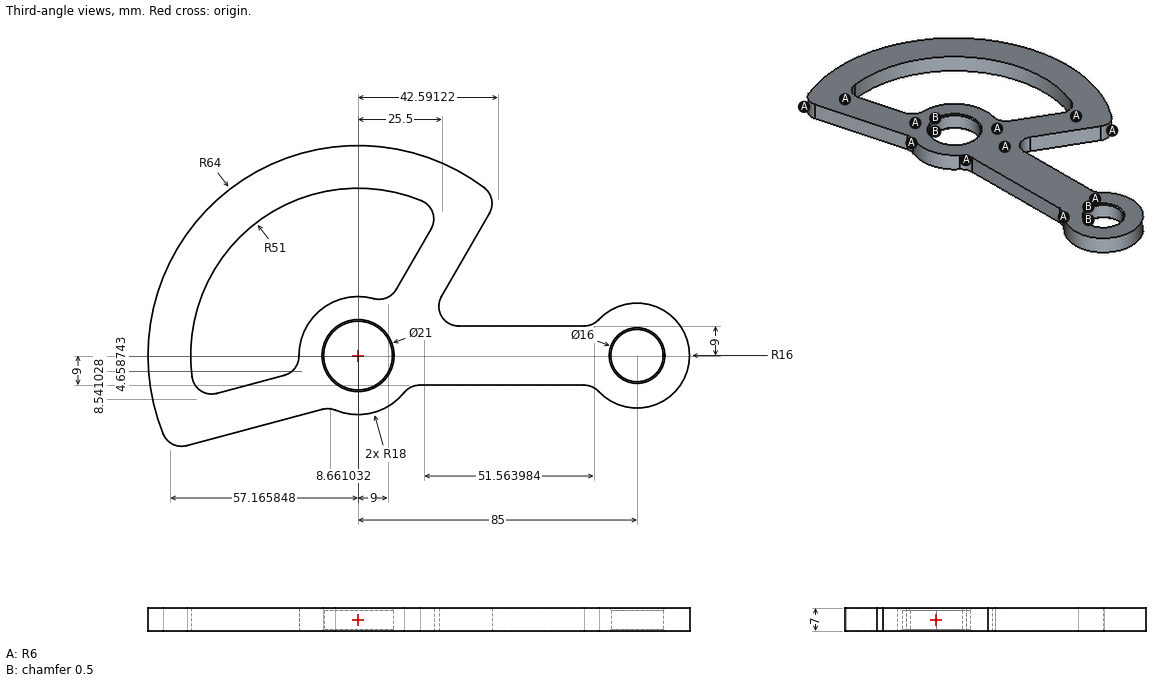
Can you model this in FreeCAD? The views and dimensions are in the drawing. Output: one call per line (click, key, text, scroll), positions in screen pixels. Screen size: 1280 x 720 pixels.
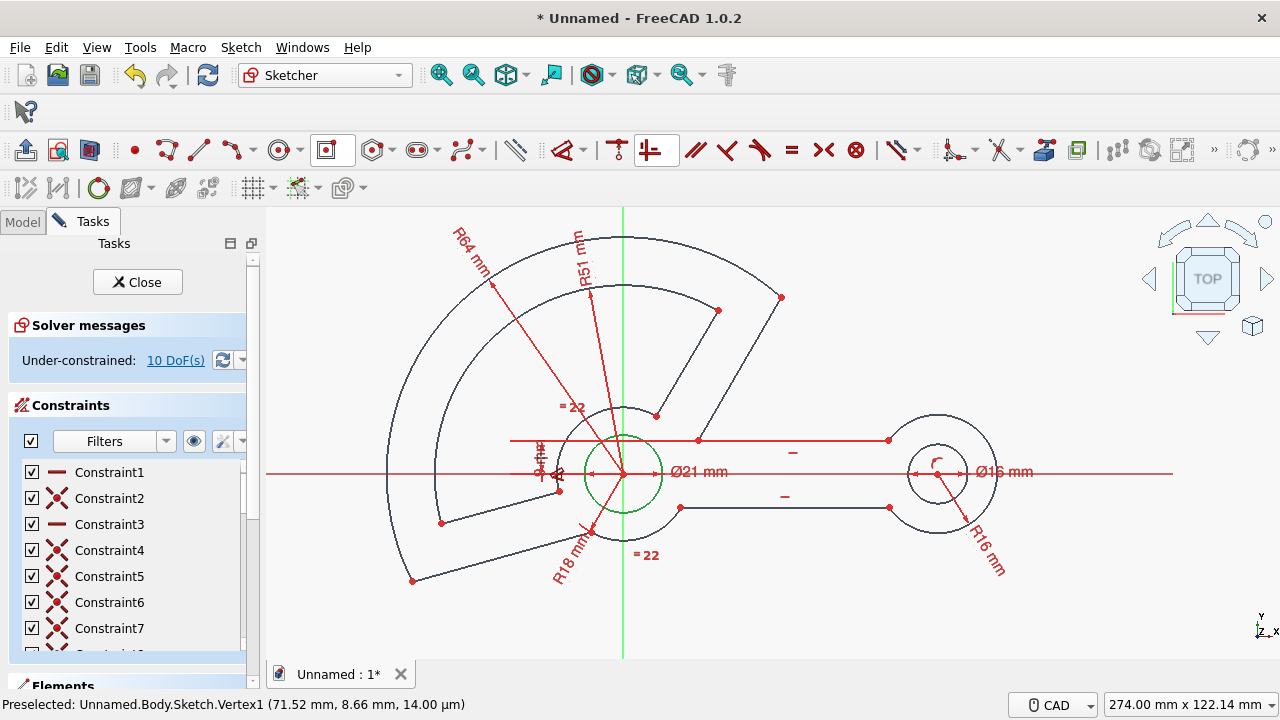
click(681, 508)
click(715, 491)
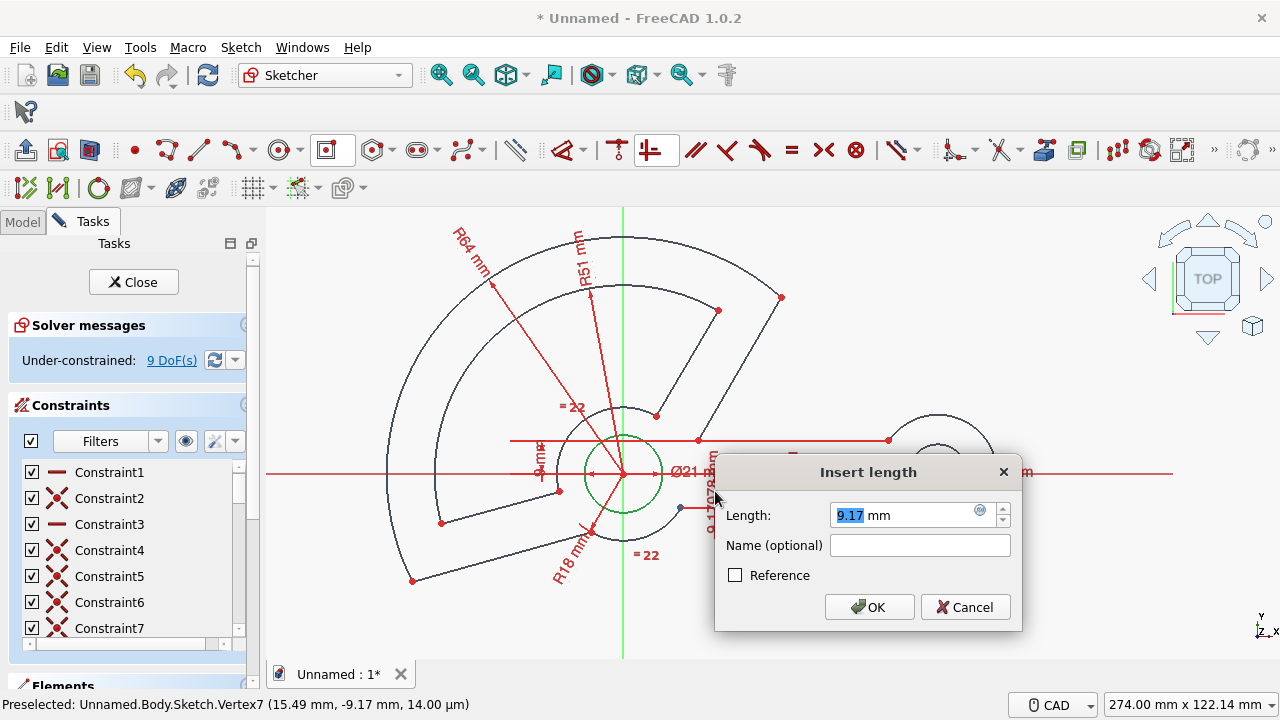
text(9)
key(Return)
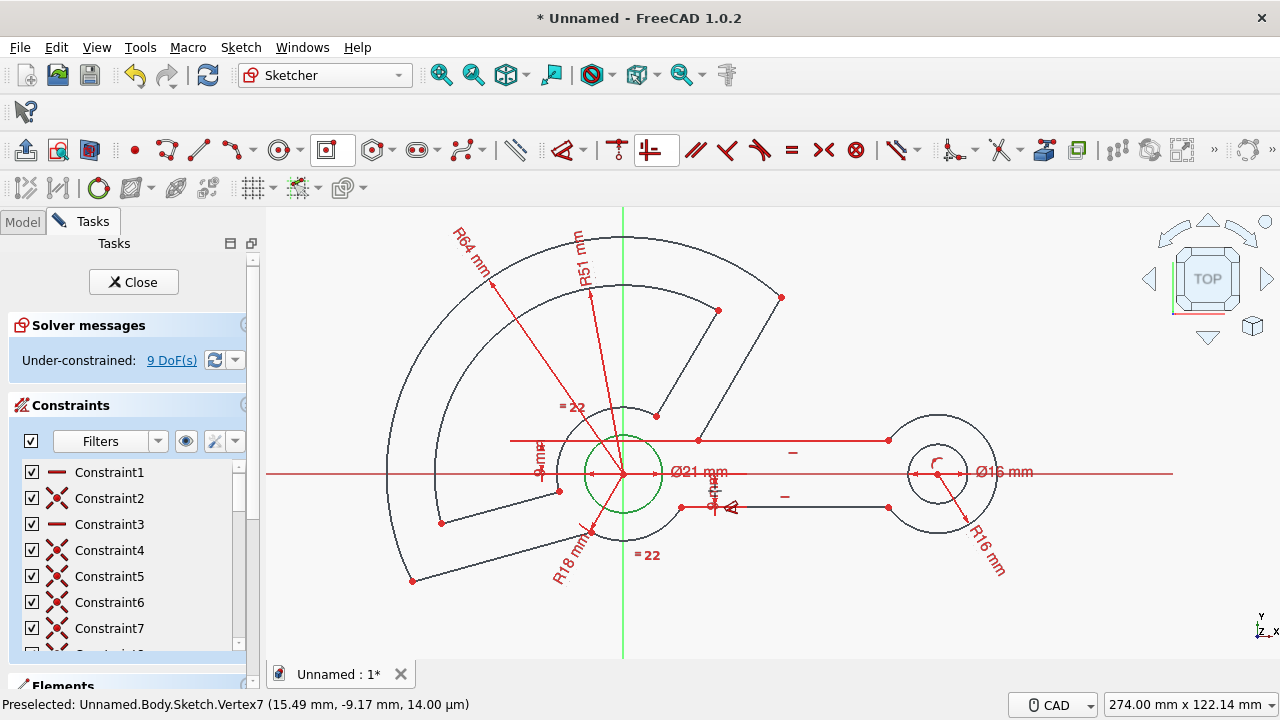
click(656, 416)
click(640, 382)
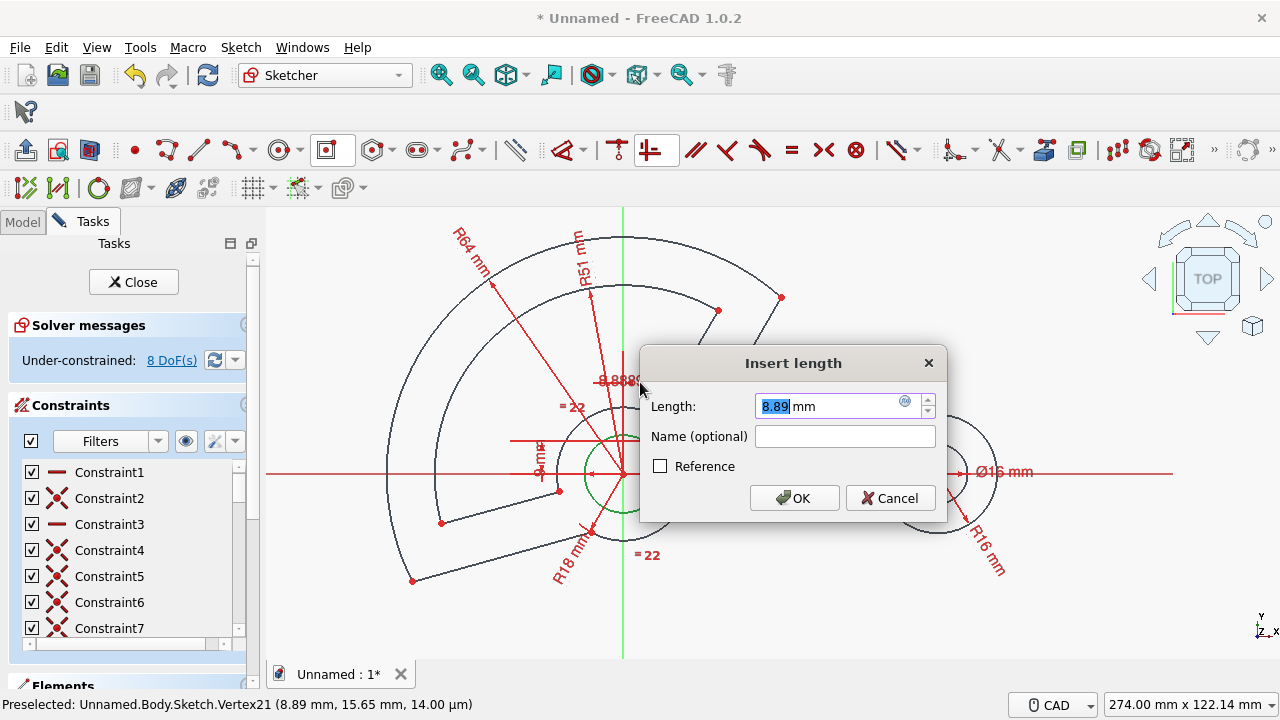
text(9)
key(Return)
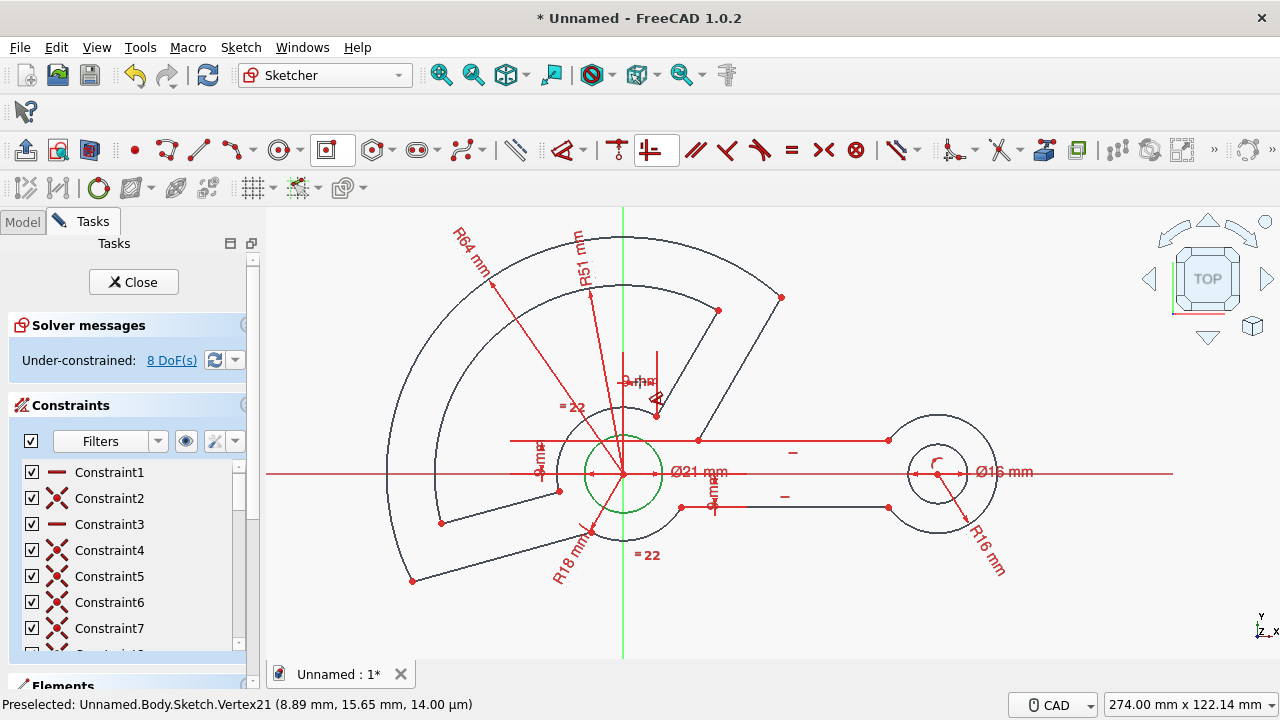
click(938, 474)
click(671, 440)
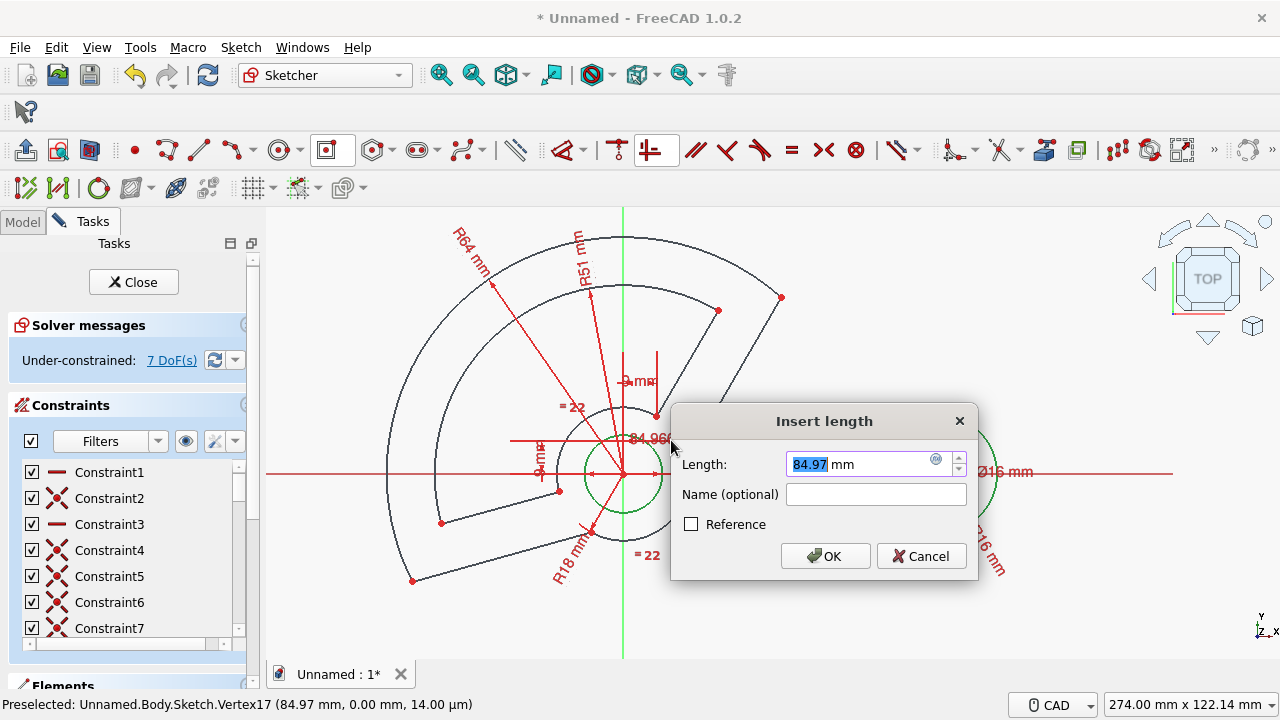
text(85)
key(Return)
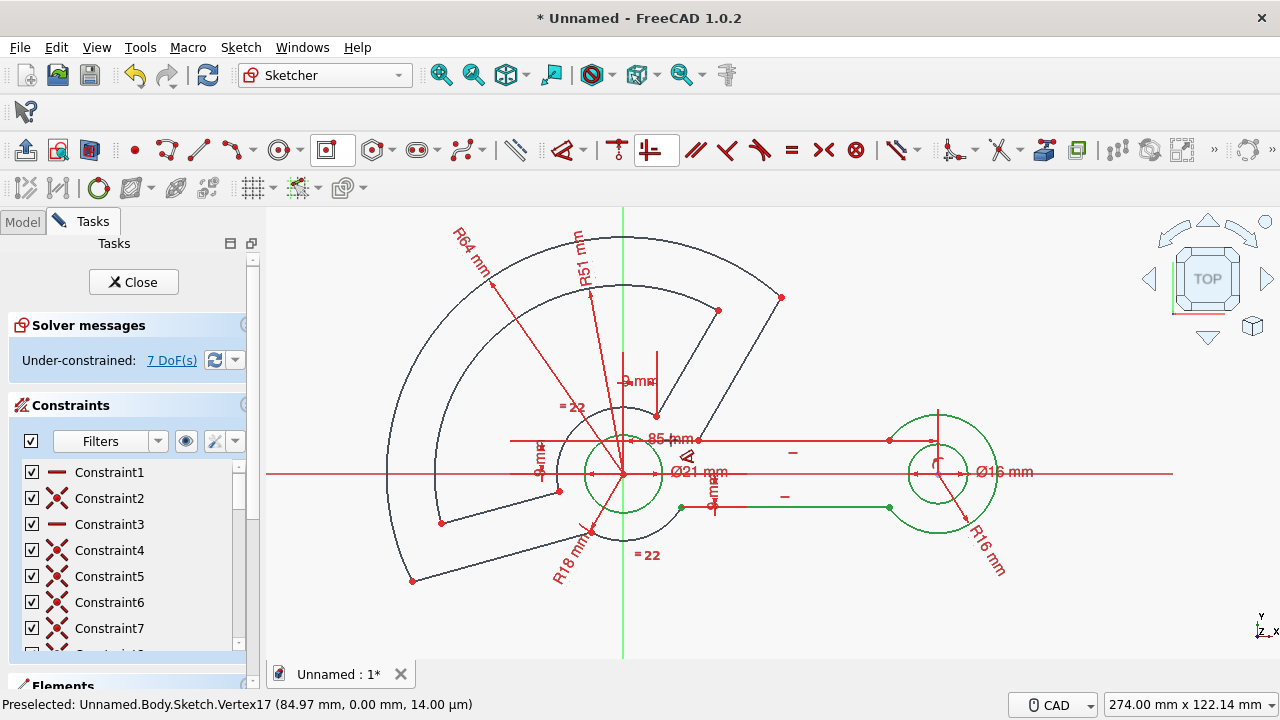
click(718, 311)
click(671, 277)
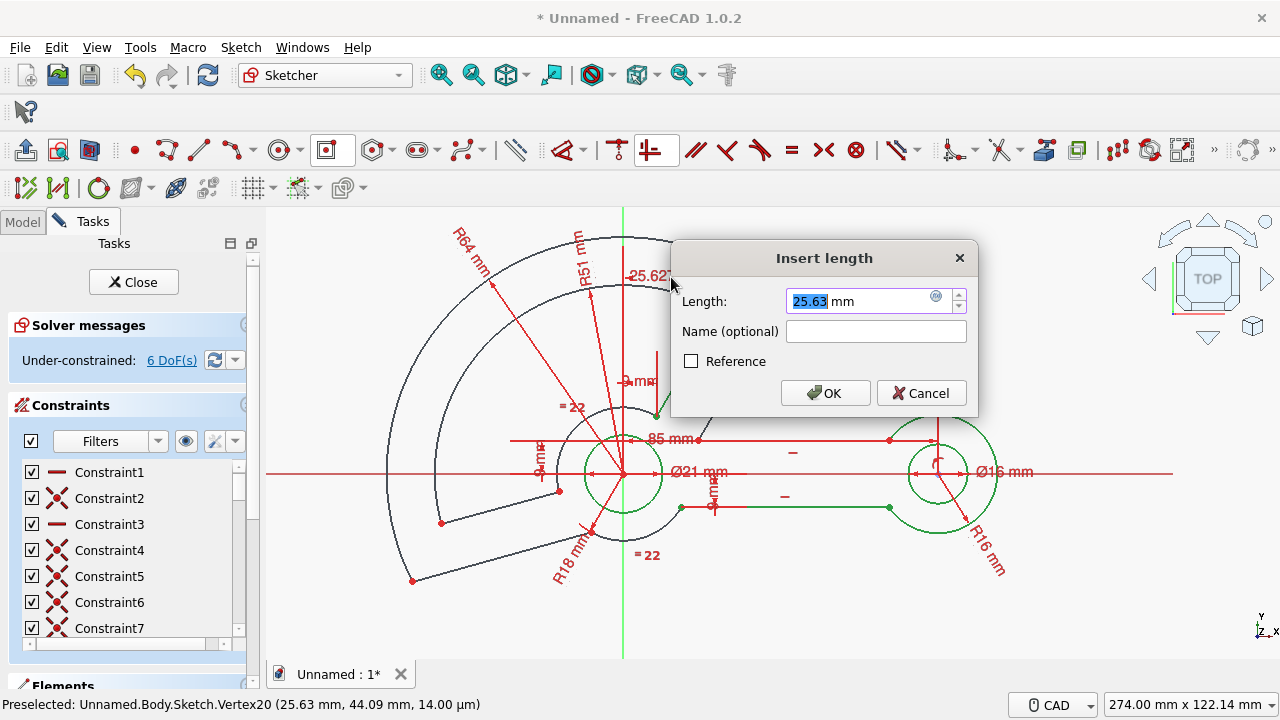
text(25.5)
key(Return)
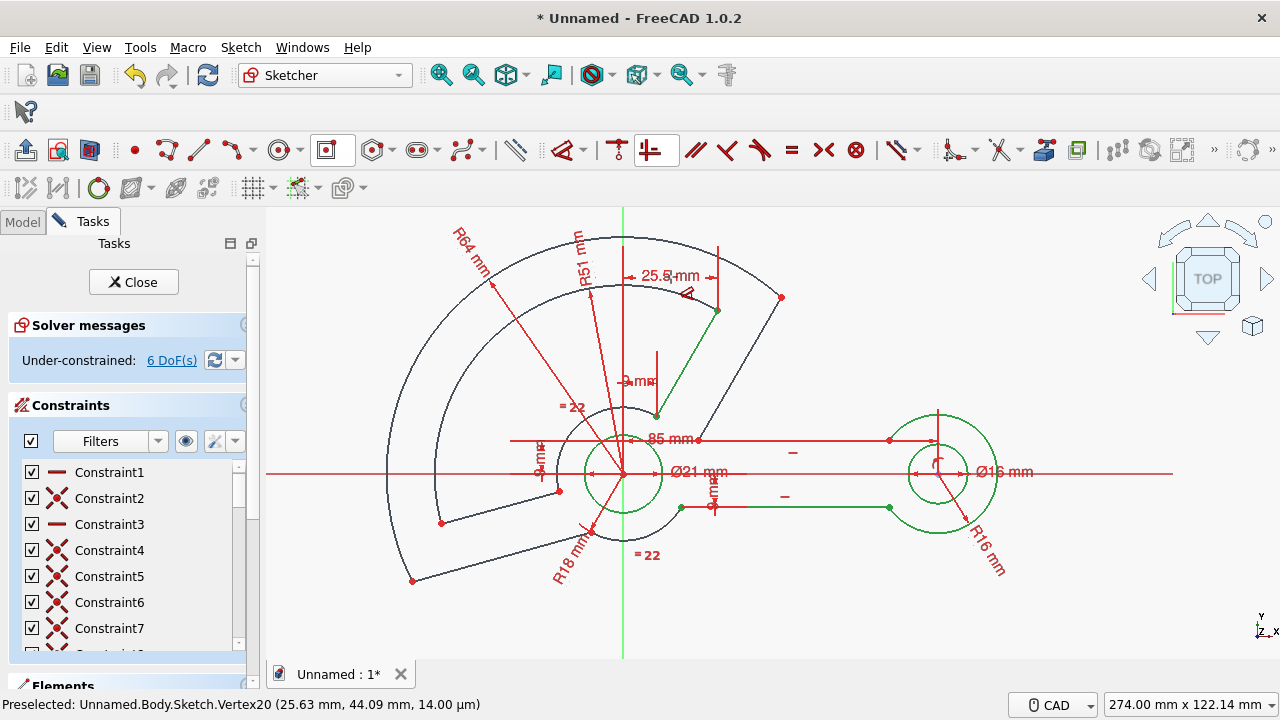
click(832, 441)
click(794, 407)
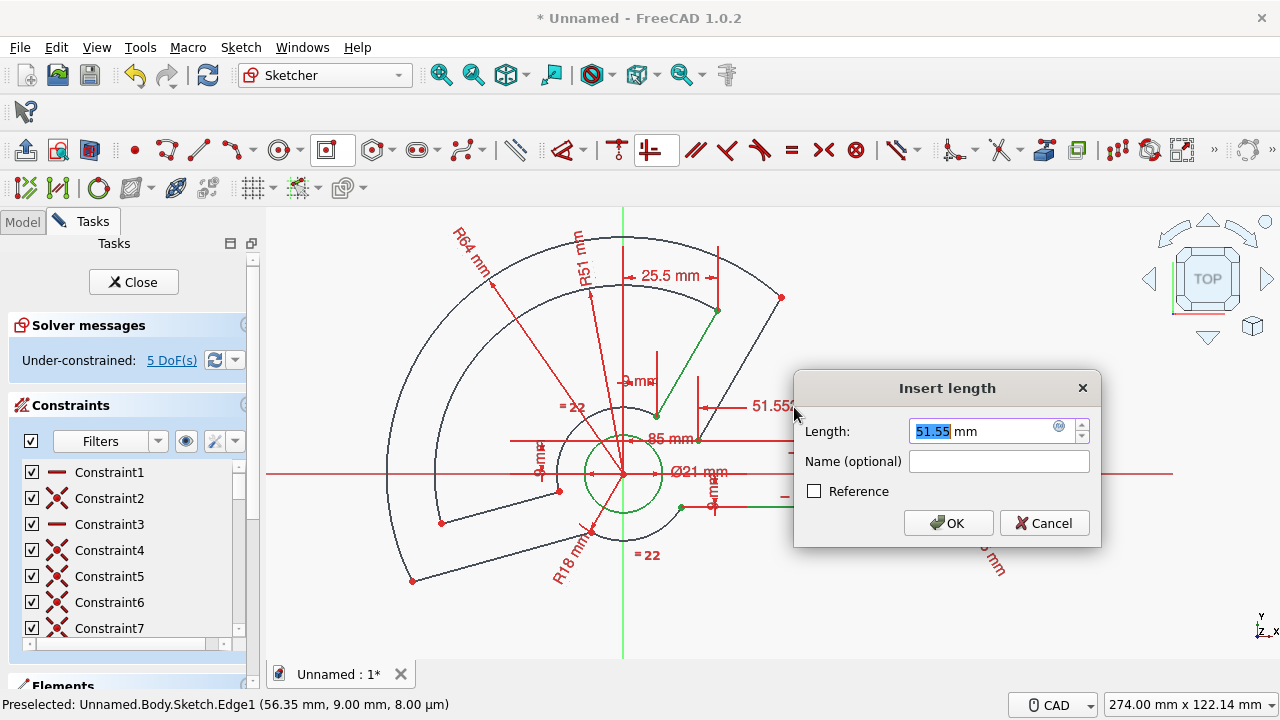
text(51.563984)
key(Return)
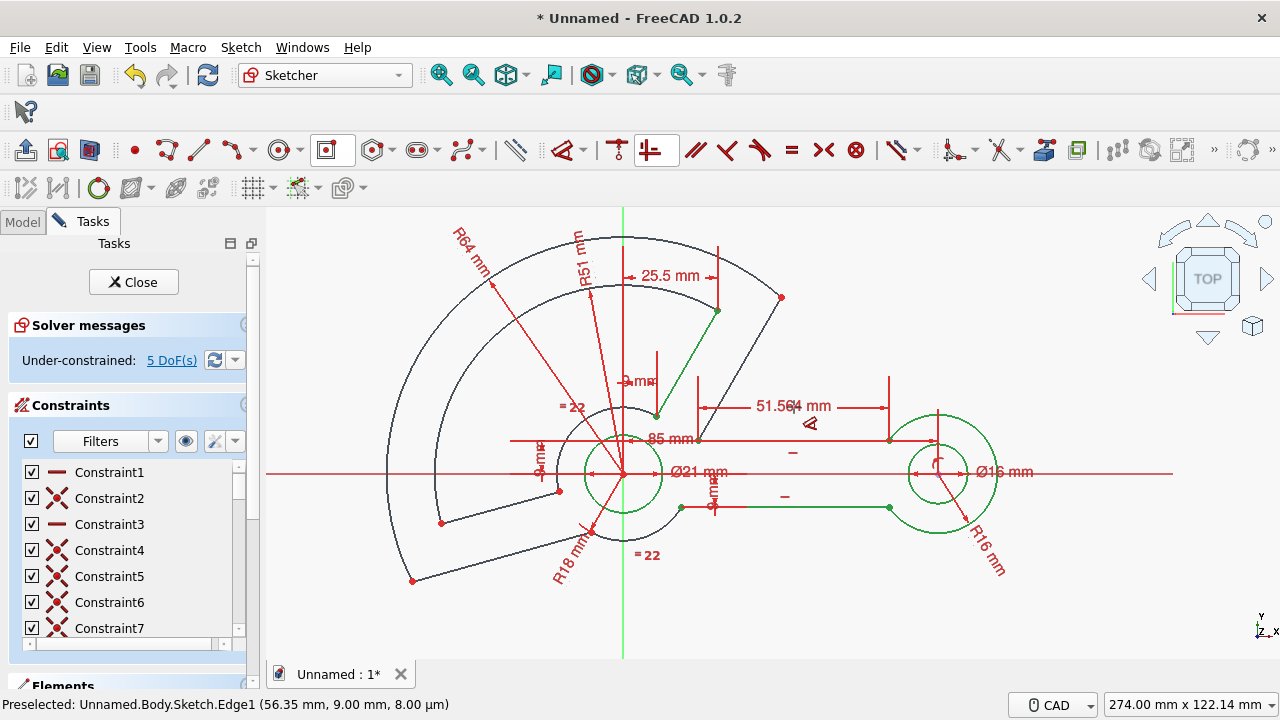
click(781, 297)
click(739, 239)